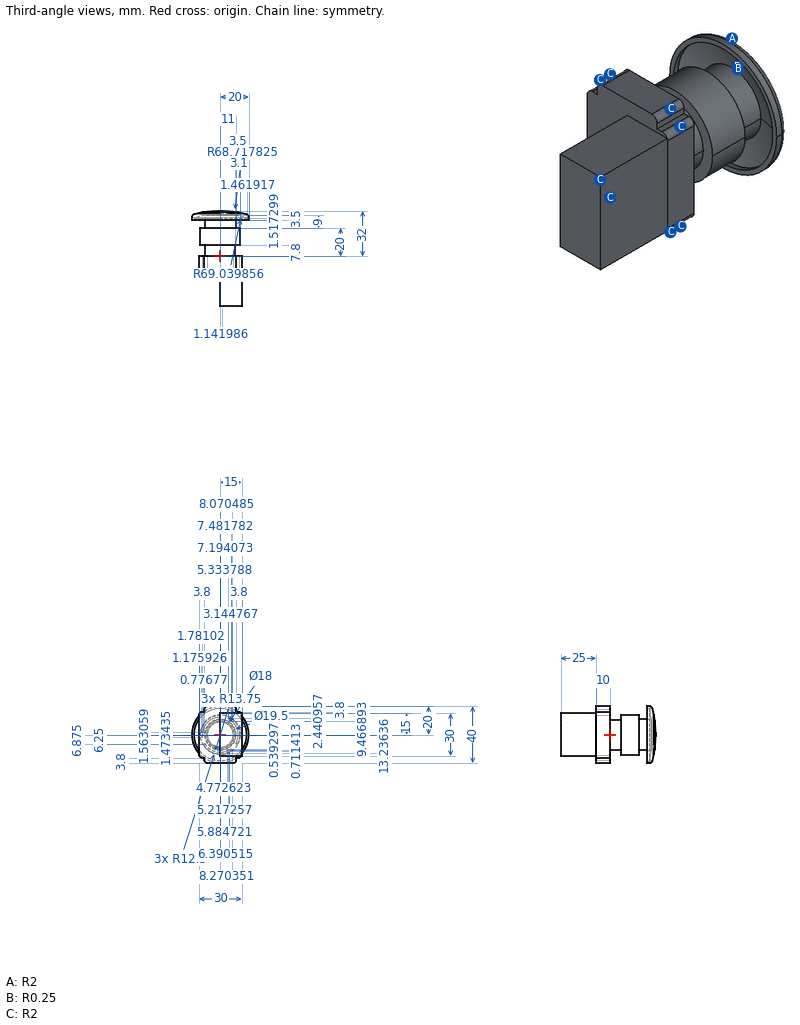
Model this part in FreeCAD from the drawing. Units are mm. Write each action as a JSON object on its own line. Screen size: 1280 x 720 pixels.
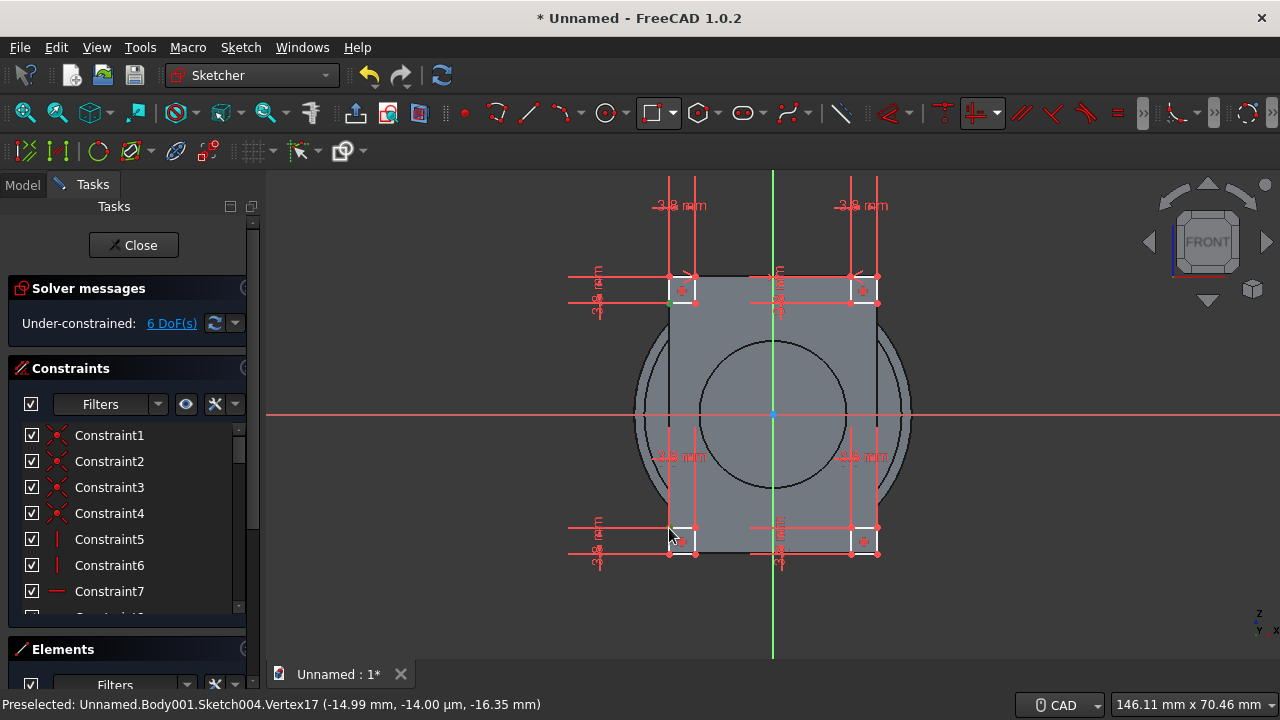
{"action": "left_click", "coordinate": [353, 414]}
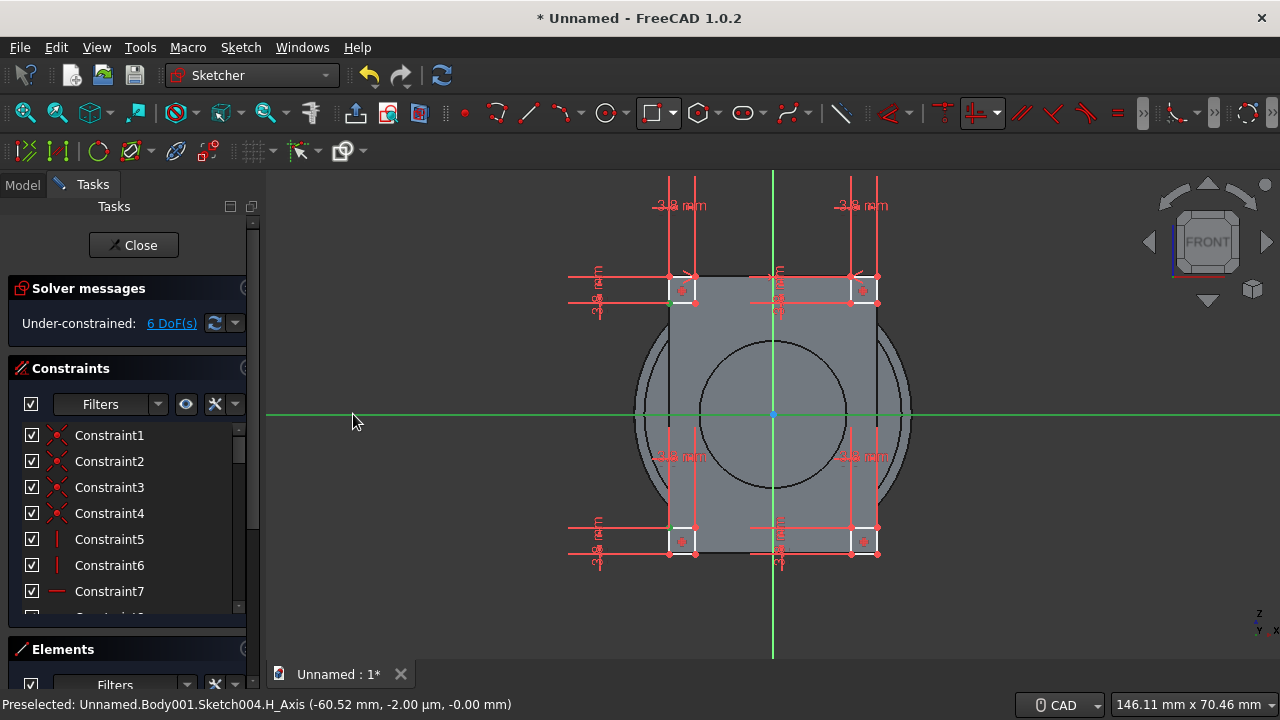
{"action": "key", "text": "s"}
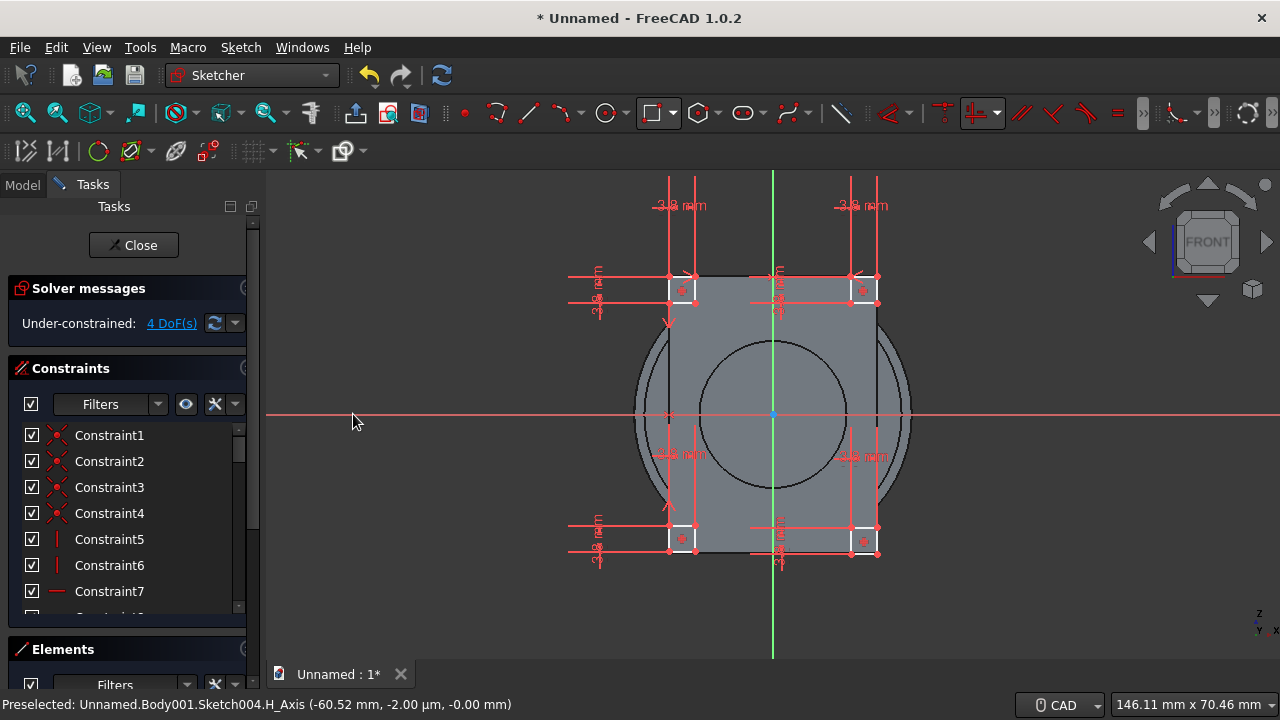
{"action": "left_click", "coordinate": [851, 303]}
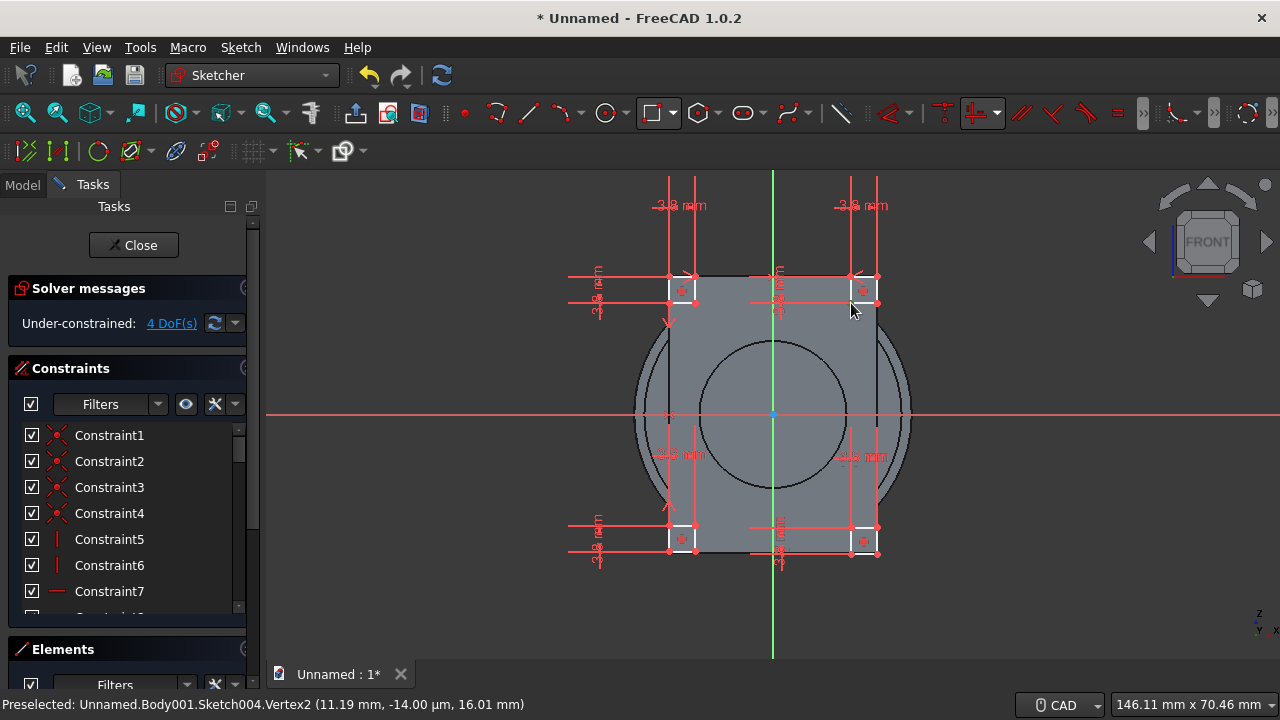
{"action": "left_click", "coordinate": [851, 528]}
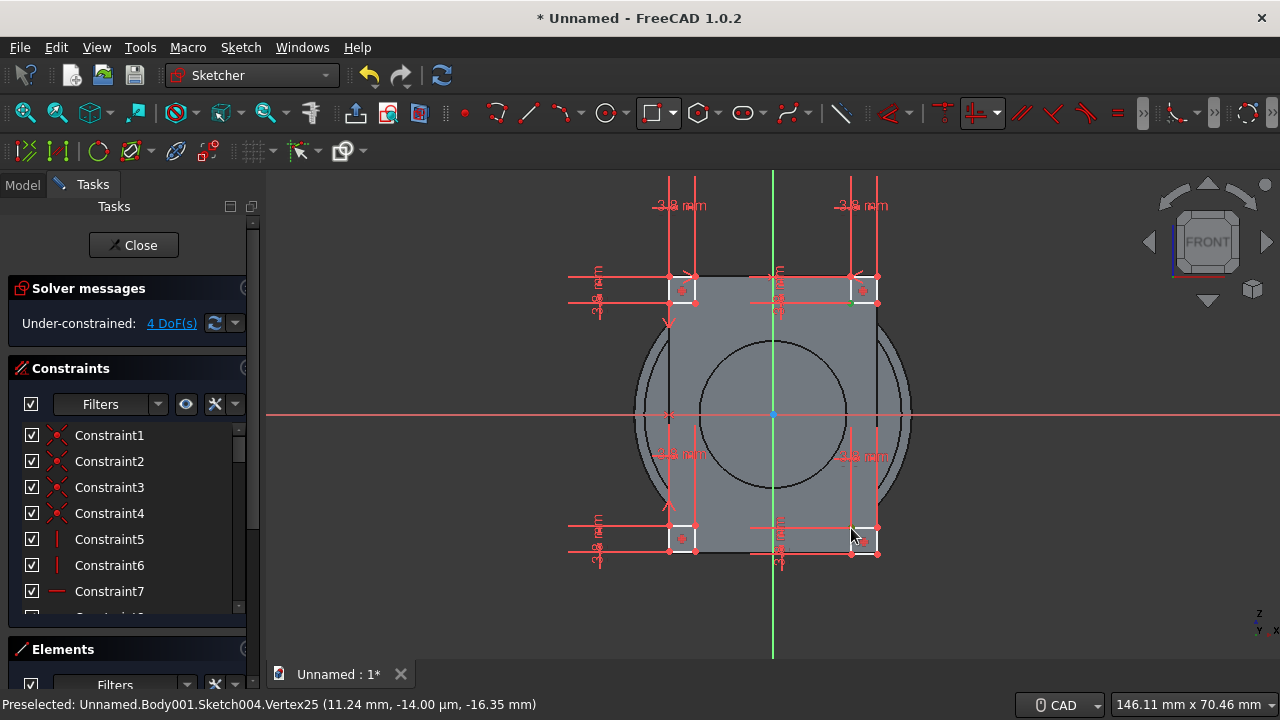
{"action": "left_click", "coordinate": [353, 414]}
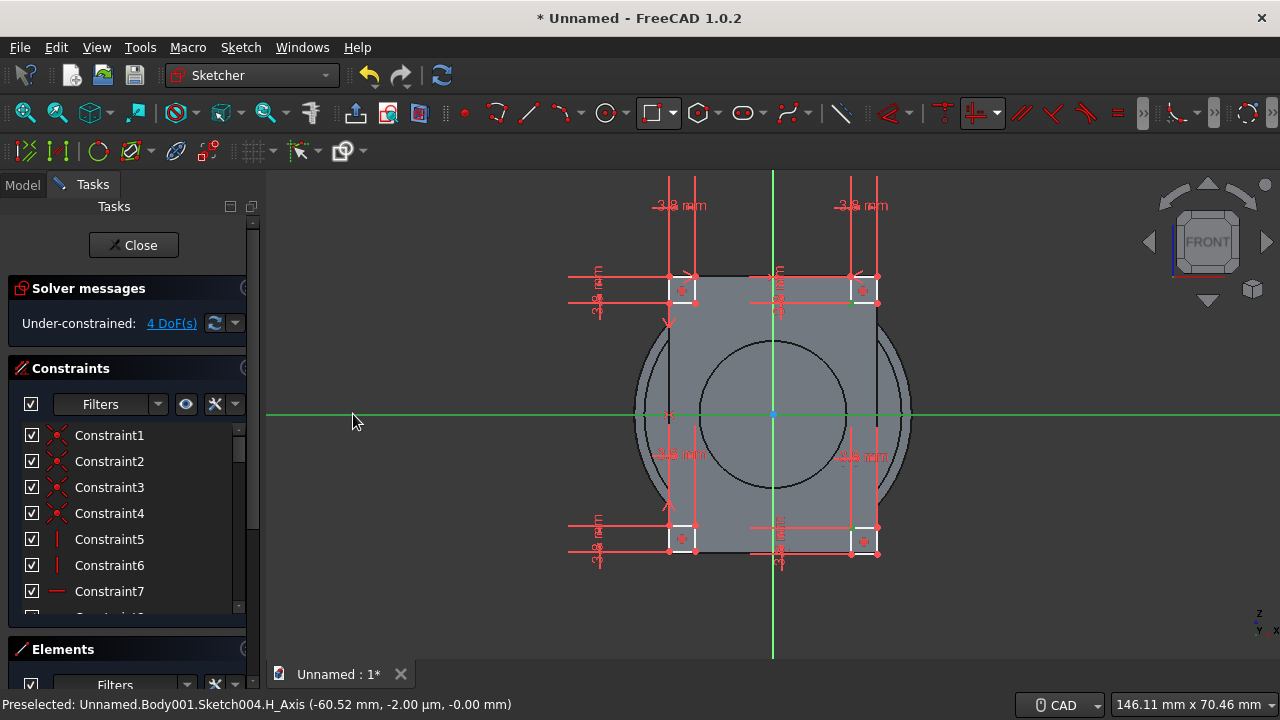
{"action": "key", "text": "s"}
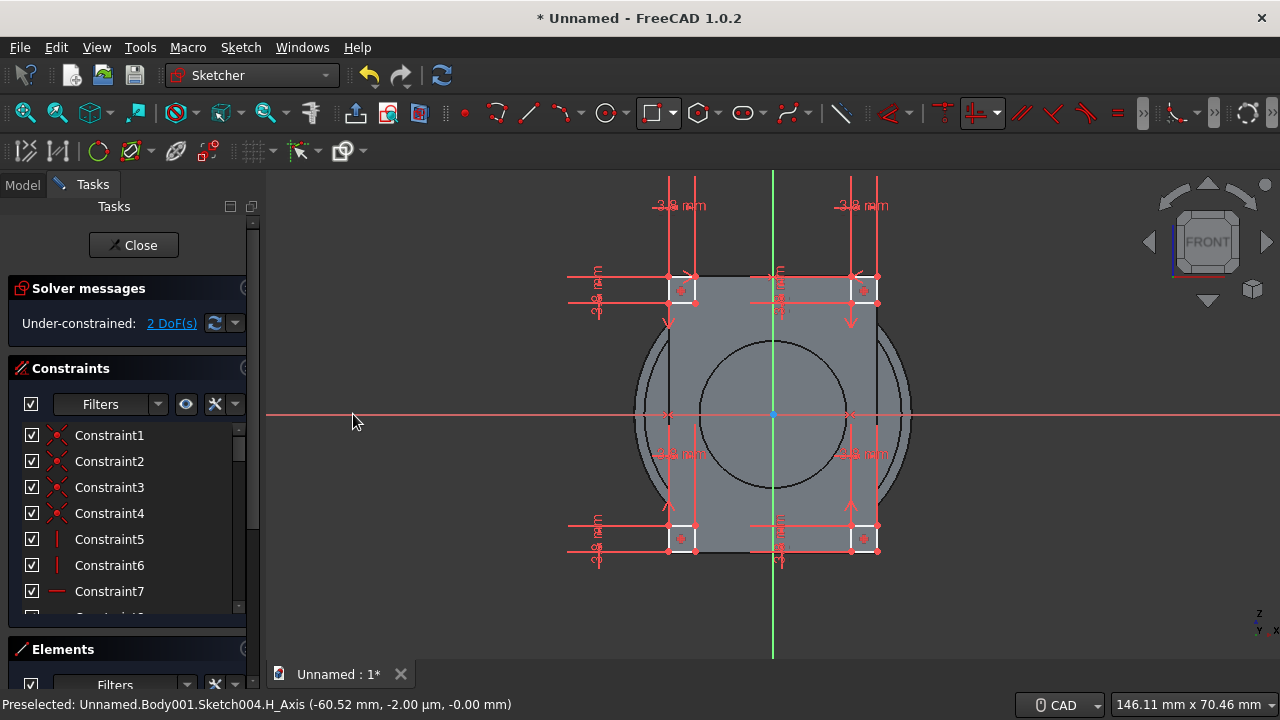
{"action": "left_click", "coordinate": [888, 114]}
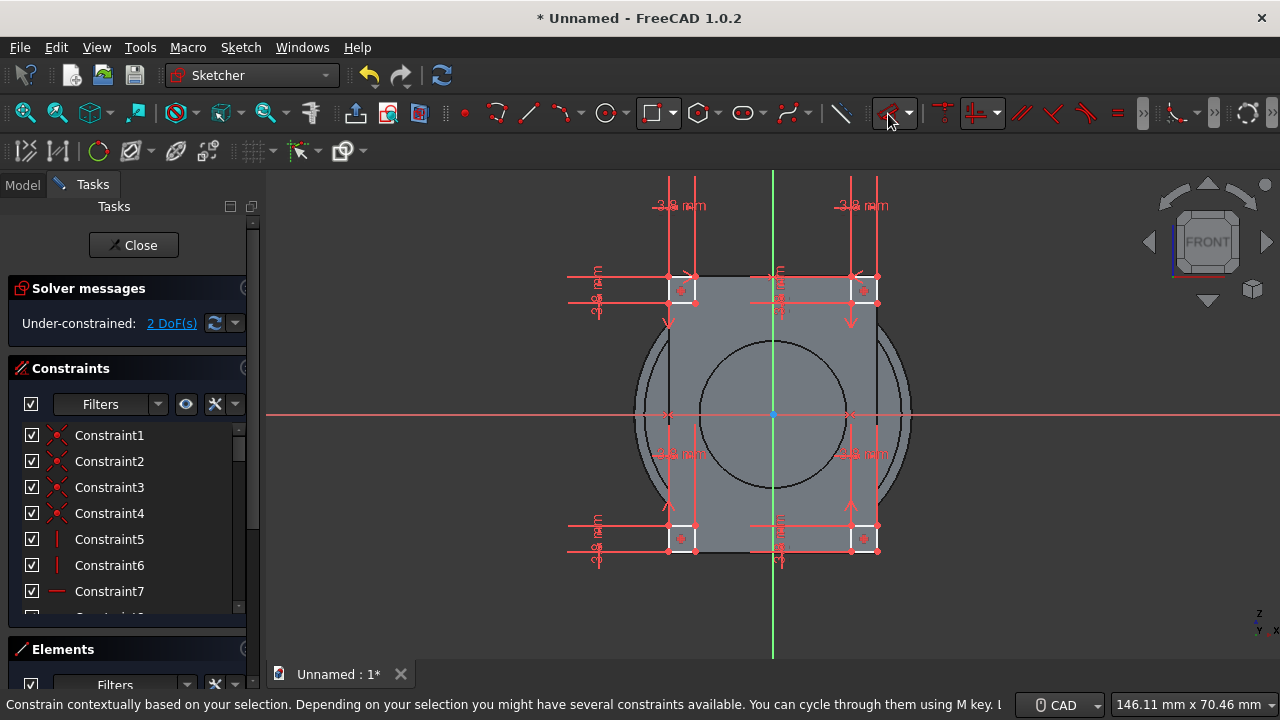
{"action": "left_click", "coordinate": [851, 277]}
{"action": "left_click", "coordinate": [885, 346]}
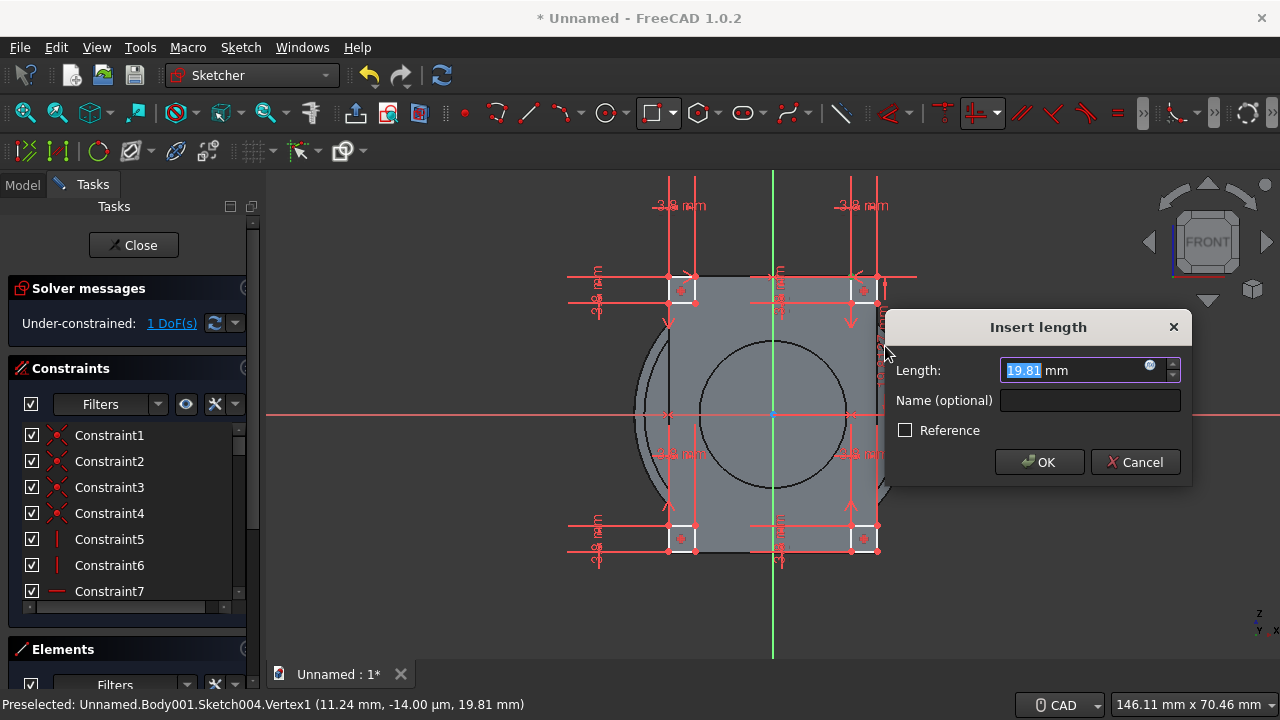
{"action": "type", "text": "20"}
{"action": "key", "text": "Return"}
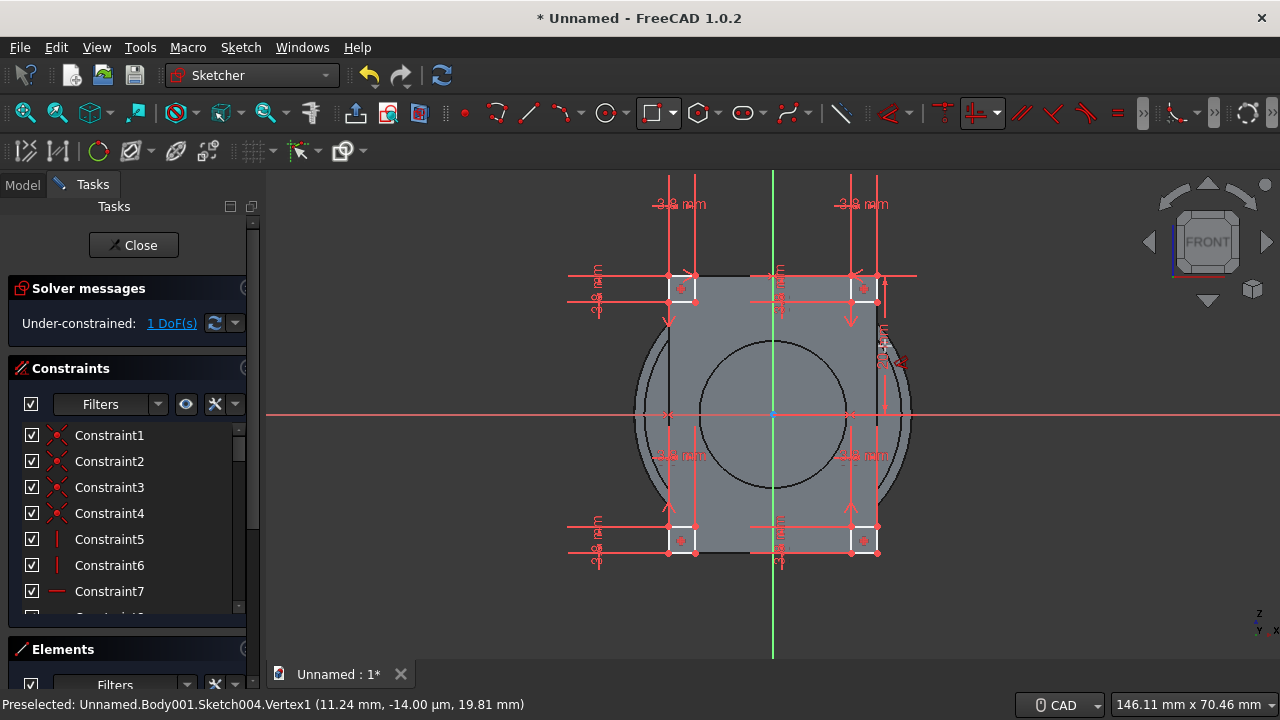
{"action": "left_click", "coordinate": [877, 302]}
{"action": "left_click", "coordinate": [825, 268]}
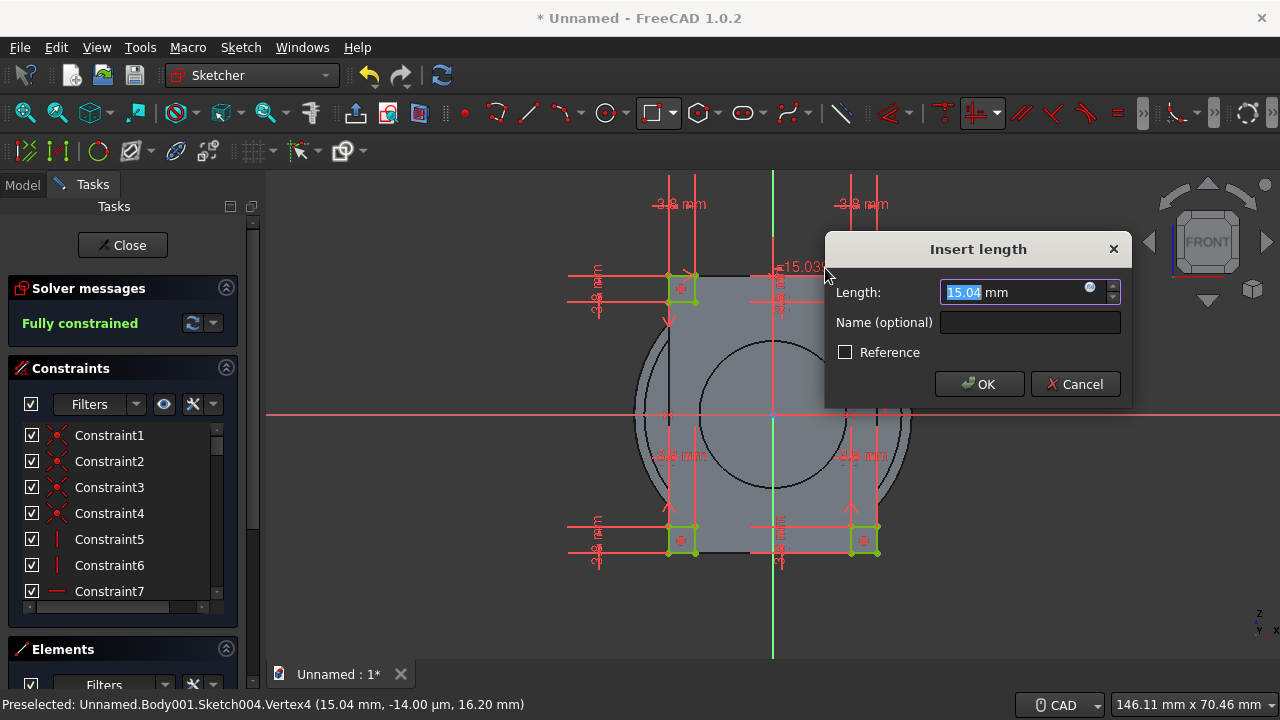
{"action": "type", "text": "15"}
{"action": "key", "text": "Return"}
{"action": "key", "text": "Escape"}